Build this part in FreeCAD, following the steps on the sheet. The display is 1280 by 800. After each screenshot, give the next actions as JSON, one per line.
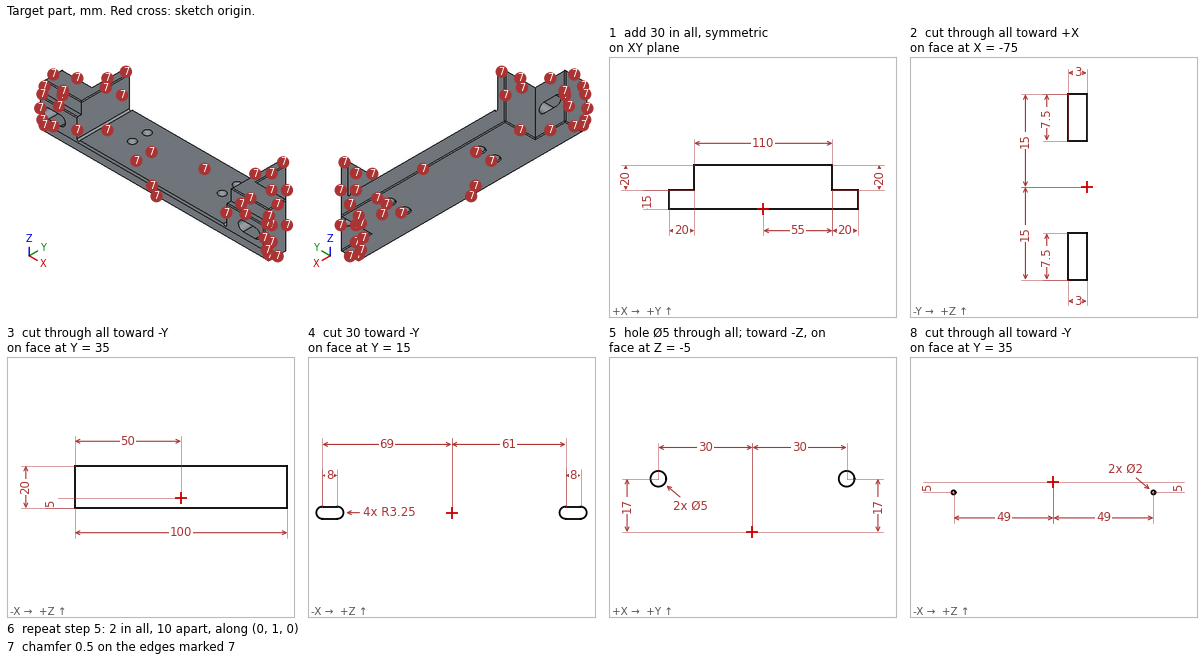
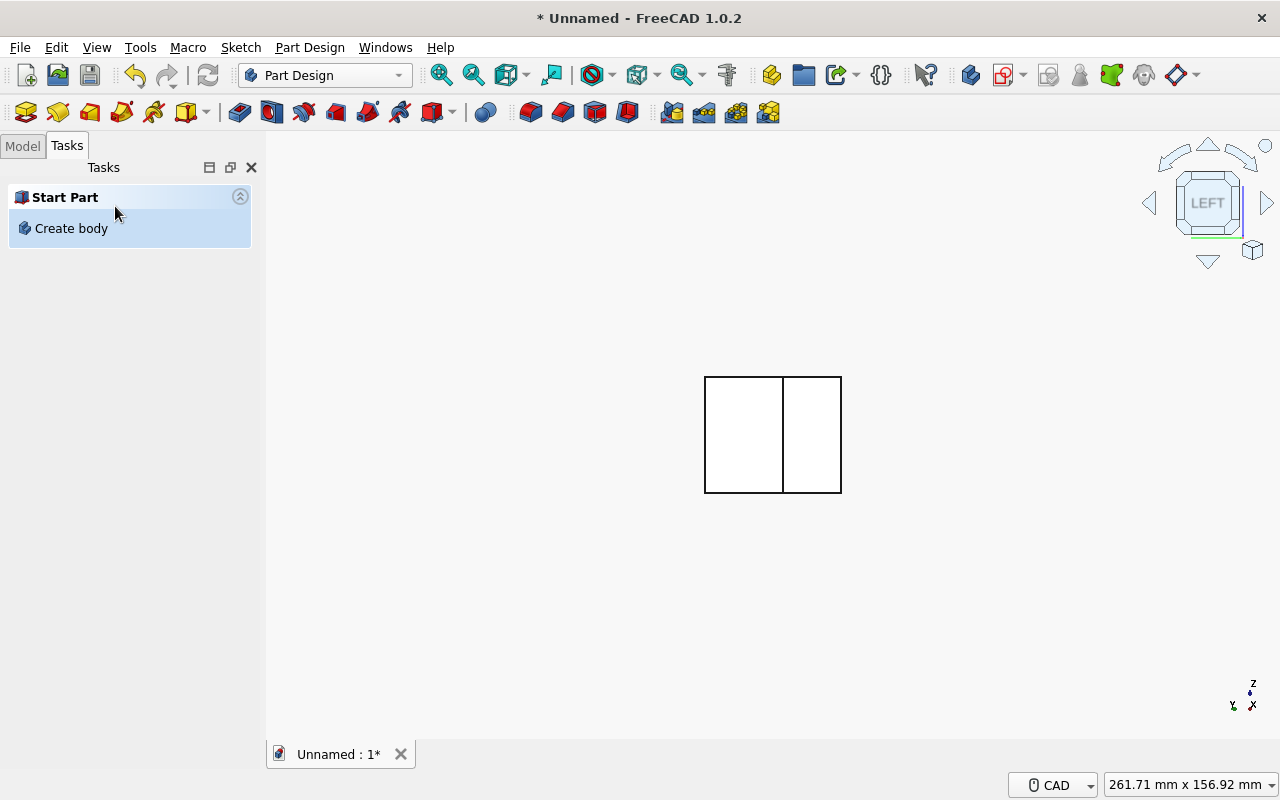
{"action": "left_click", "coordinate": [812, 417]}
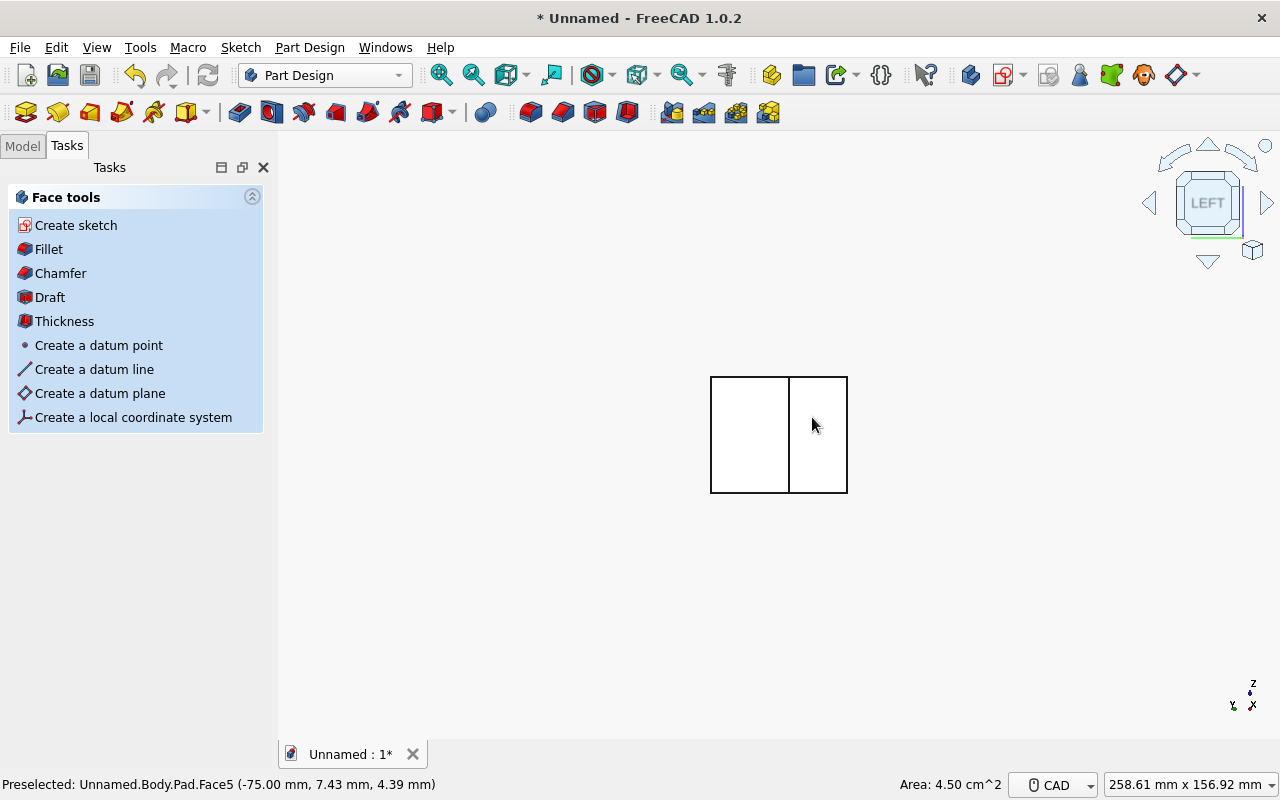
{"action": "left_click", "coordinate": [1004, 76]}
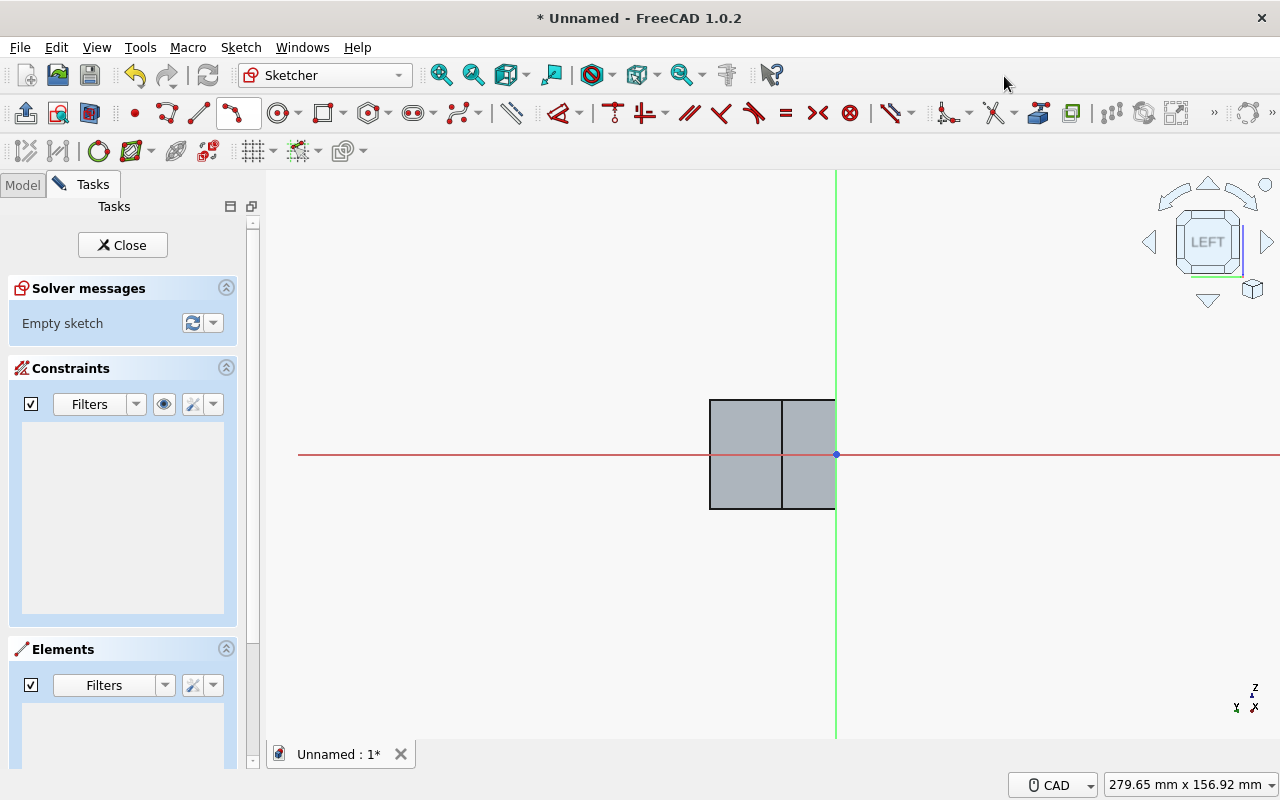
{"action": "scroll", "coordinate": [886, 455], "scroll_direction": "up", "scroll_amount": 6}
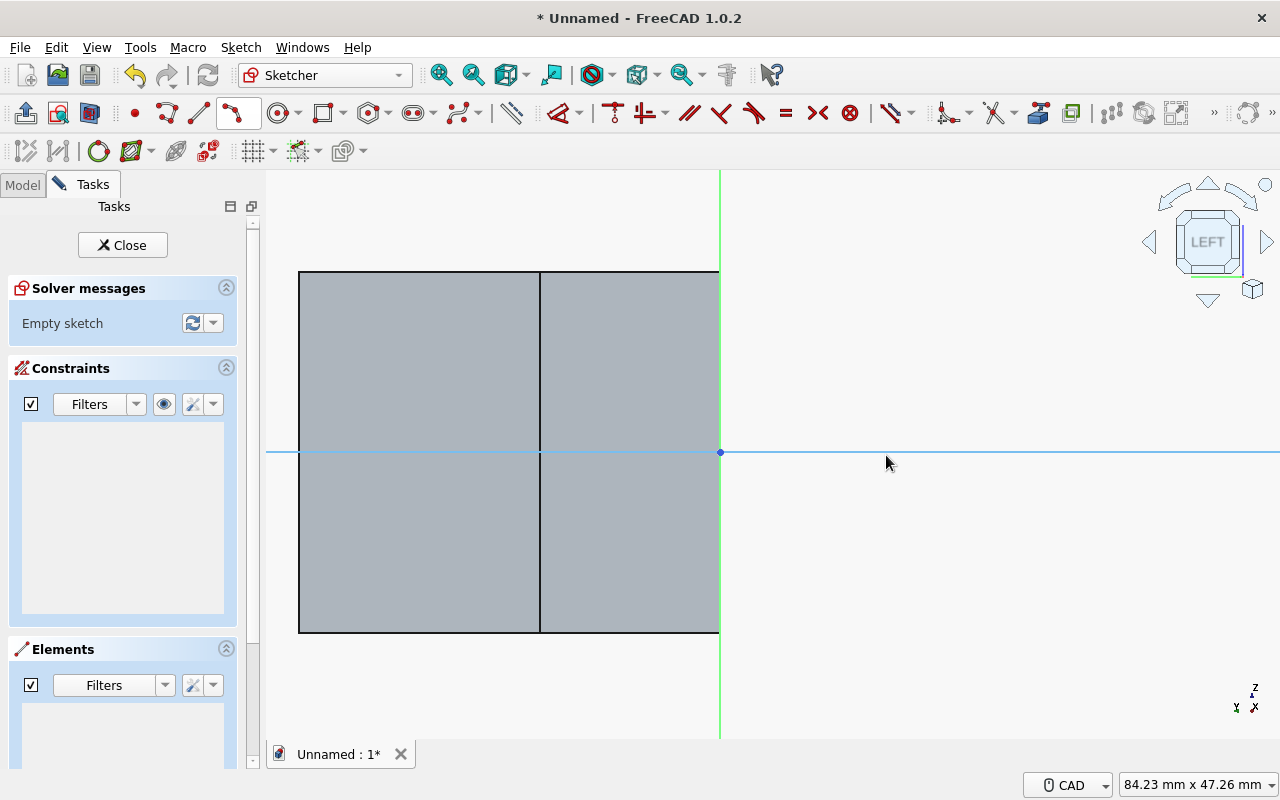
{"action": "left_click", "coordinate": [324, 114]}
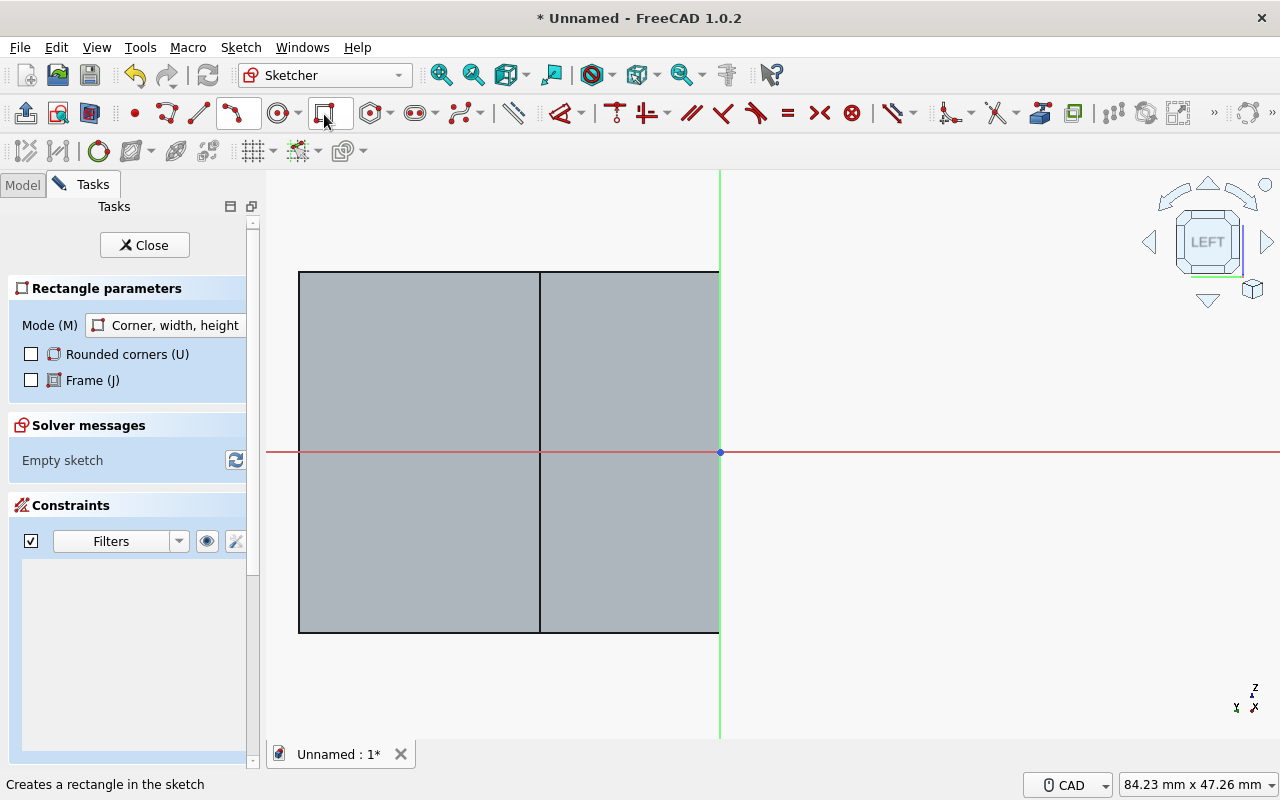
{"action": "left_click", "coordinate": [684, 542]}
{"action": "left_click", "coordinate": [720, 633]}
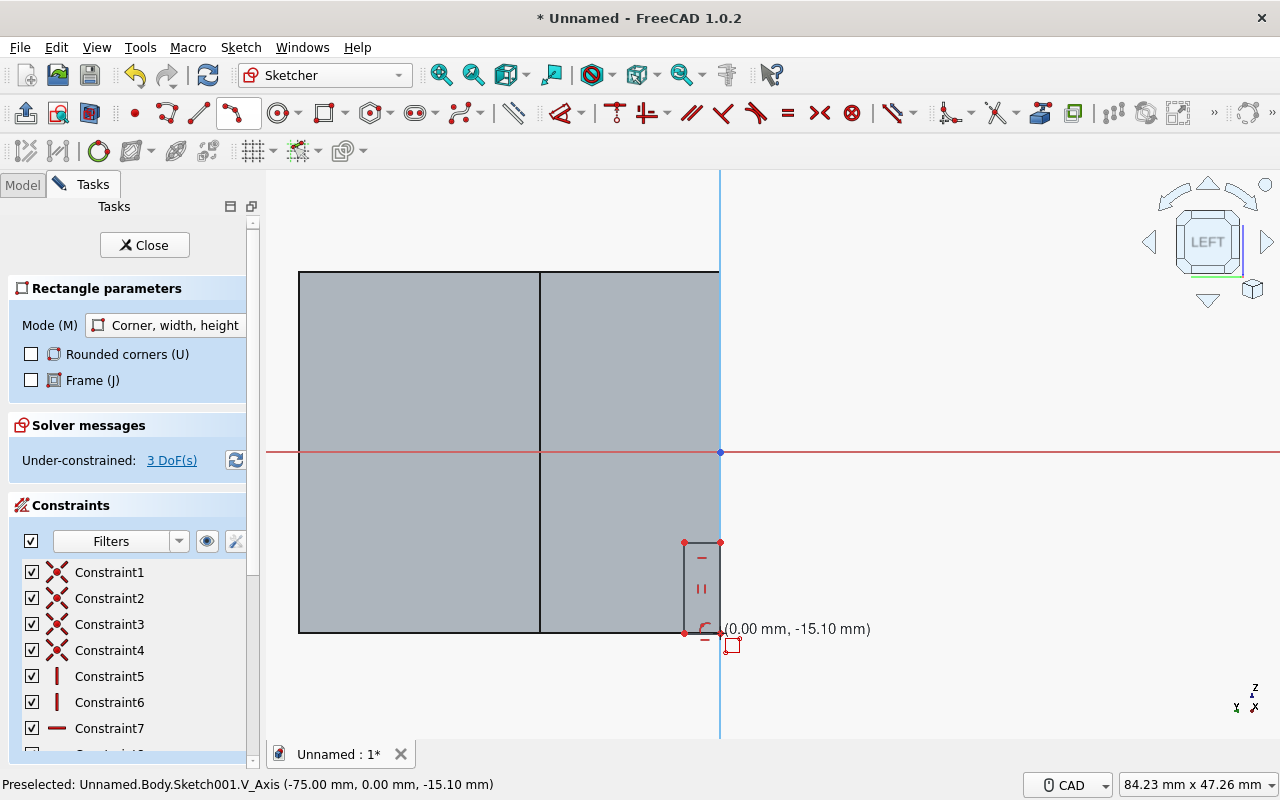
{"action": "left_click", "coordinate": [684, 272]}
{"action": "left_click", "coordinate": [720, 362]}
{"action": "key", "text": "Escape"}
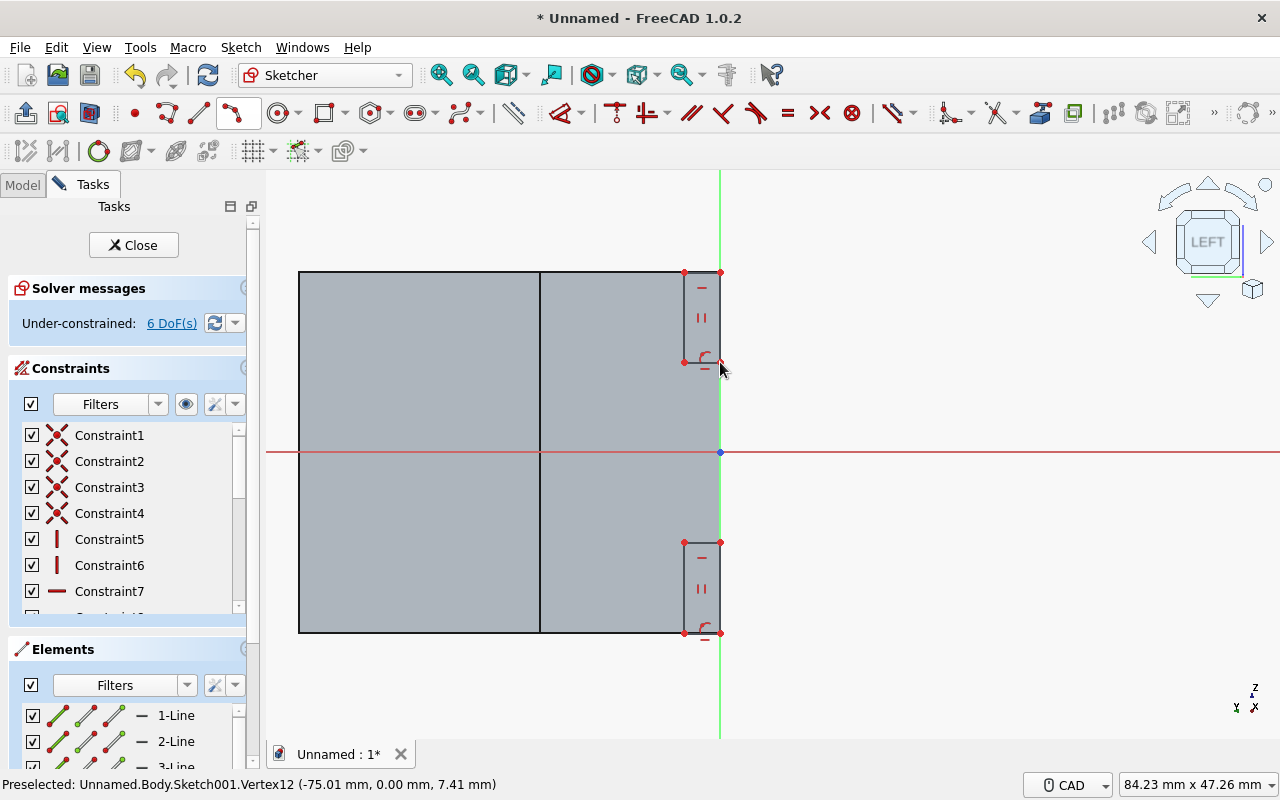
{"action": "key", "text": "d"}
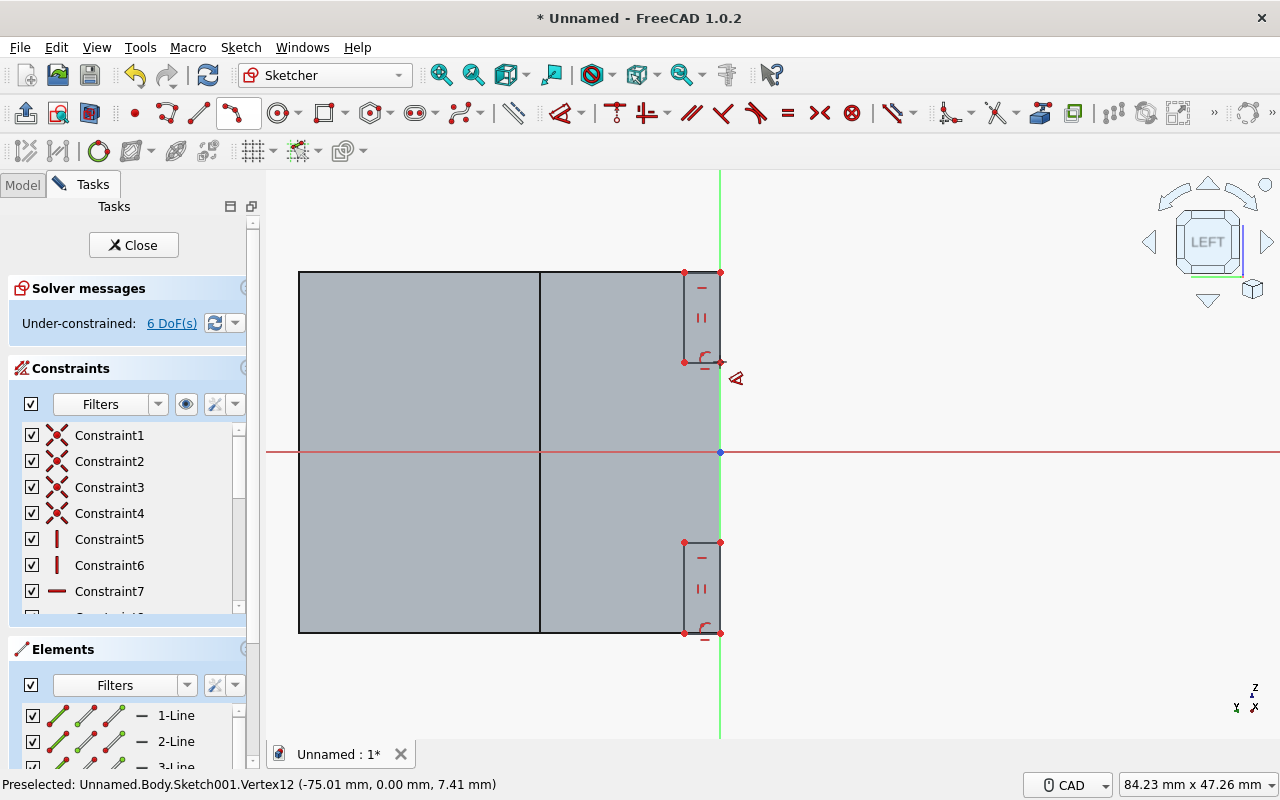
{"action": "scroll", "coordinate": [695, 634], "scroll_direction": "up", "scroll_amount": 2}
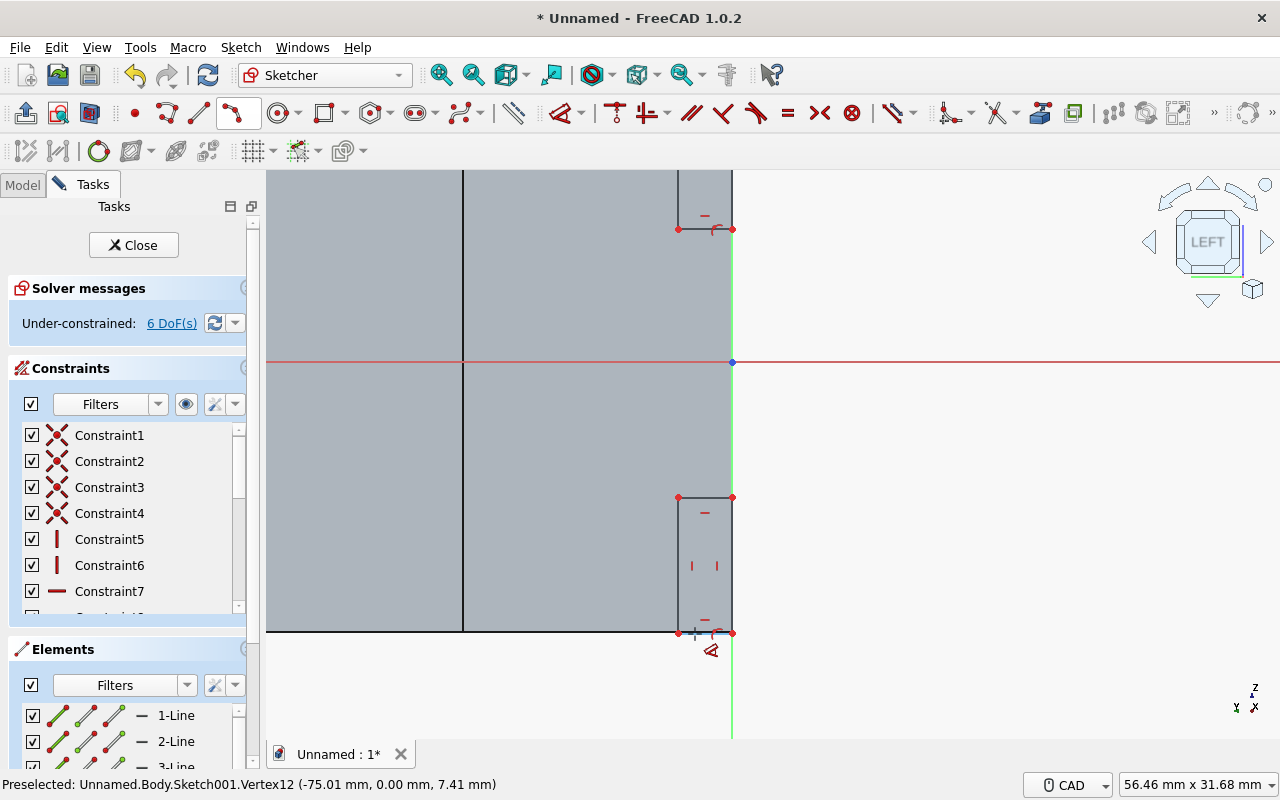
{"action": "left_click", "coordinate": [695, 634]}
{"action": "left_click", "coordinate": [705, 668]}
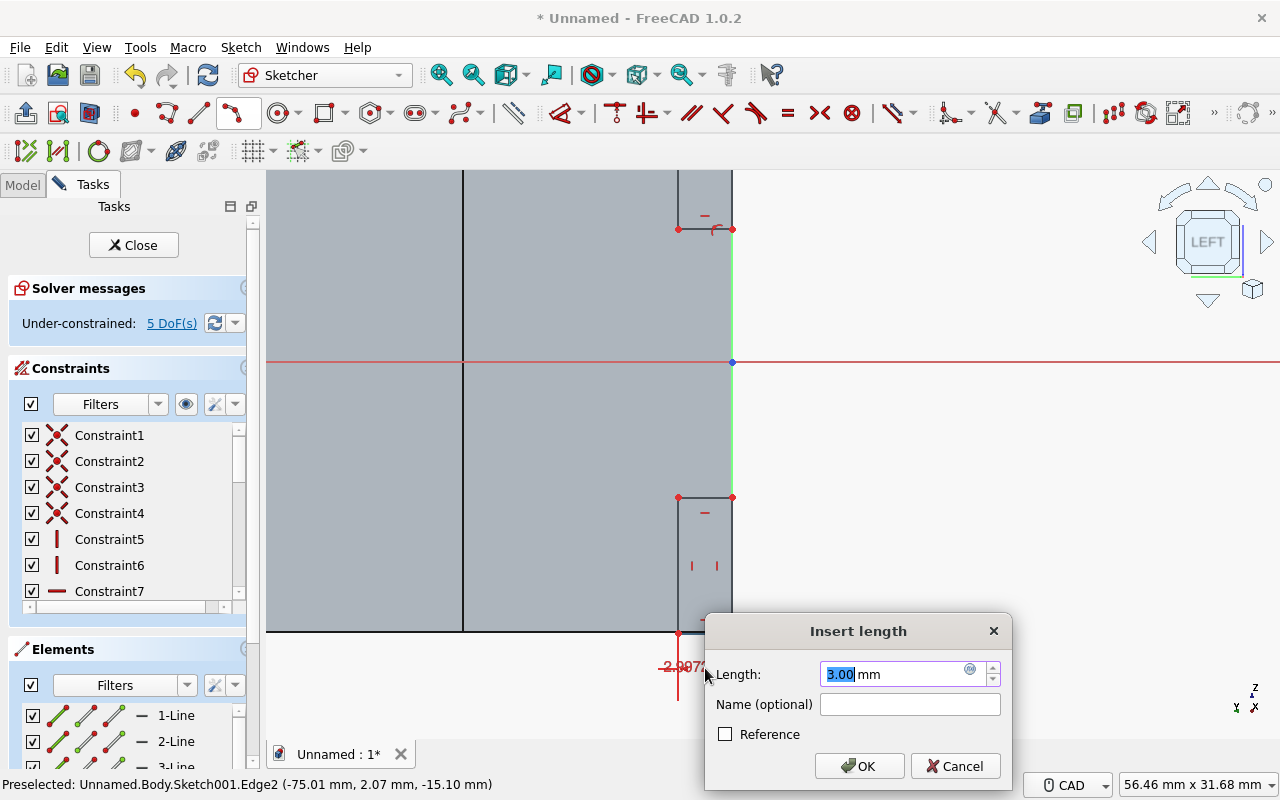
{"action": "type", "text": "3"}
{"action": "key", "text": "Return"}